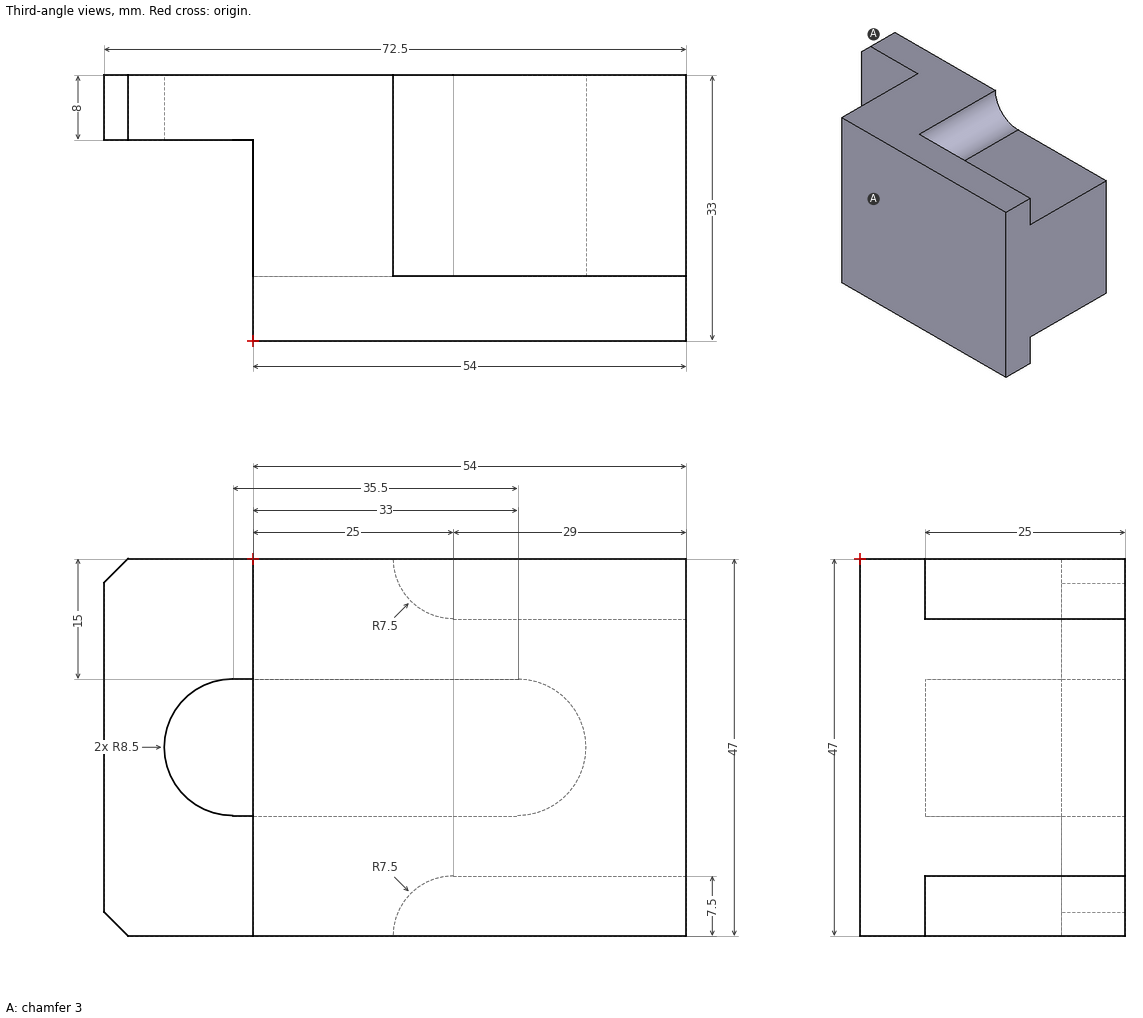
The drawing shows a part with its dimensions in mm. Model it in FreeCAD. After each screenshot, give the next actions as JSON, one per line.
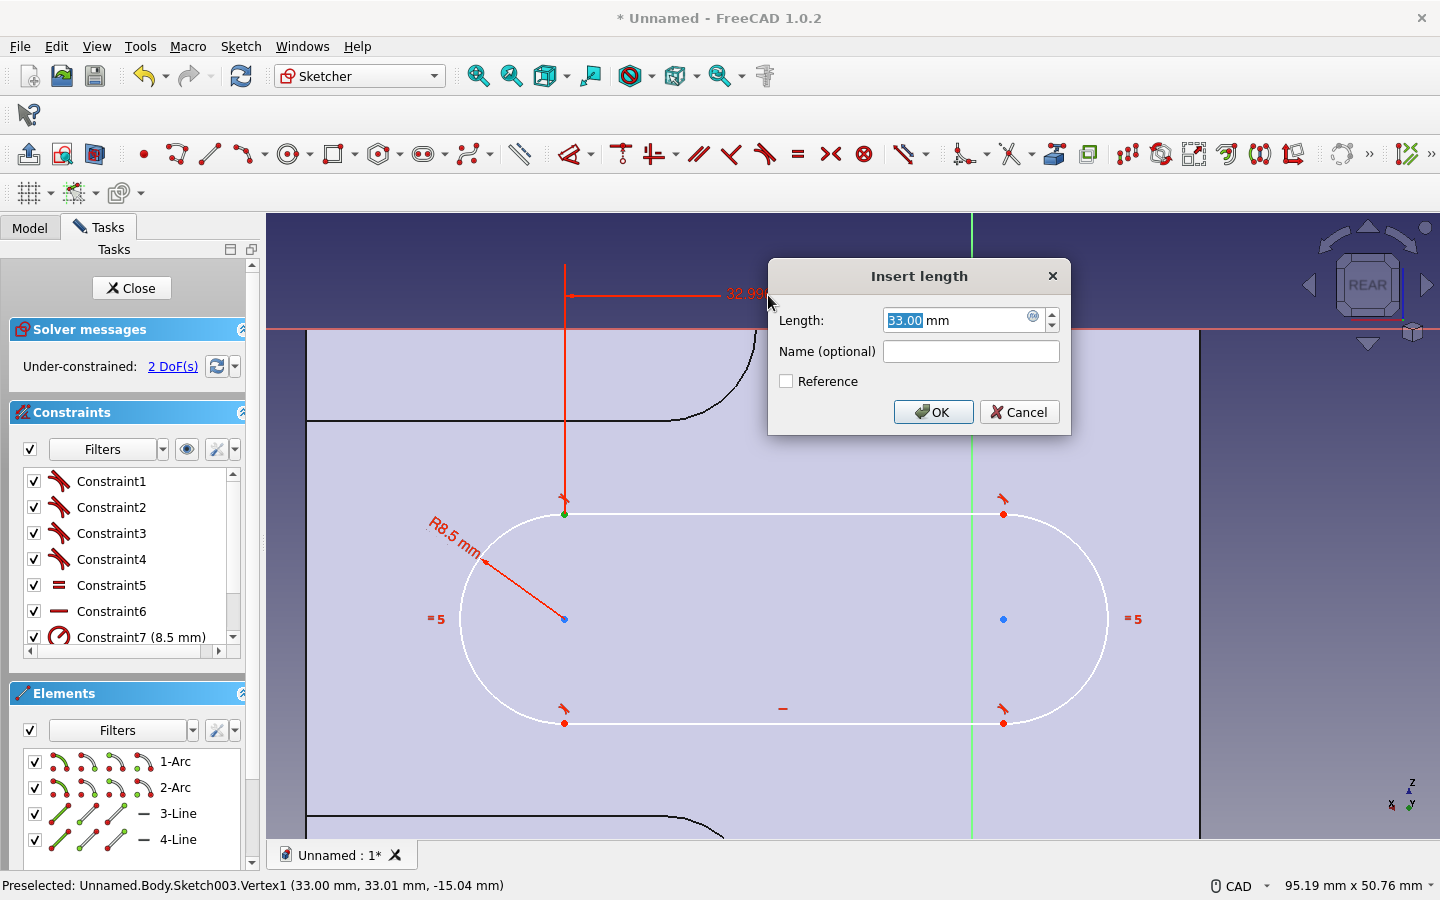
{"action": "type", "text": "33"}
{"action": "key", "text": "Return"}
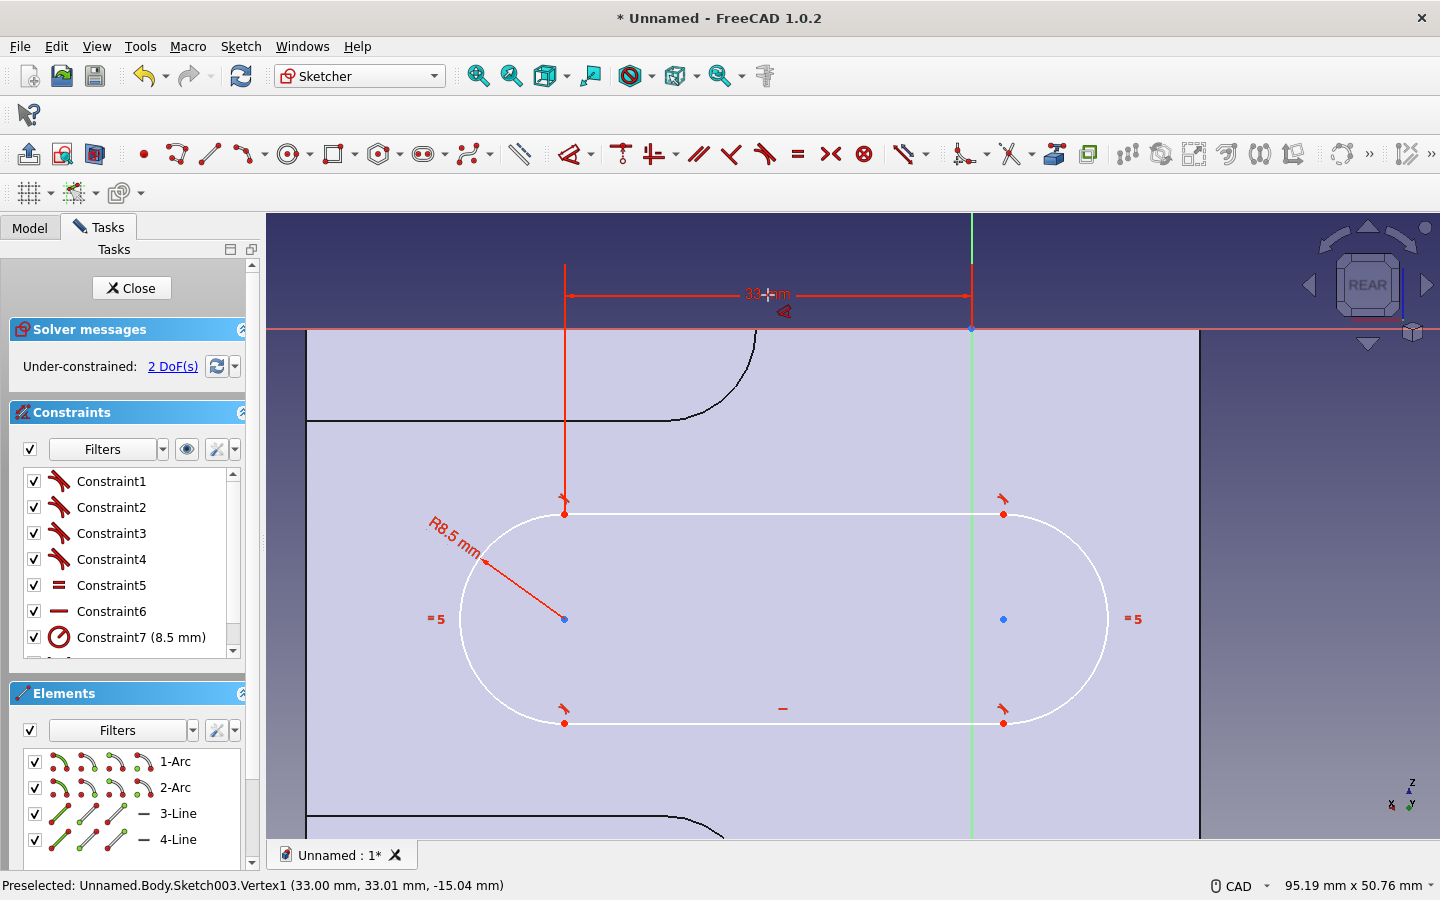
{"action": "left_click", "coordinate": [565, 514]}
{"action": "left_click", "coordinate": [531, 422]}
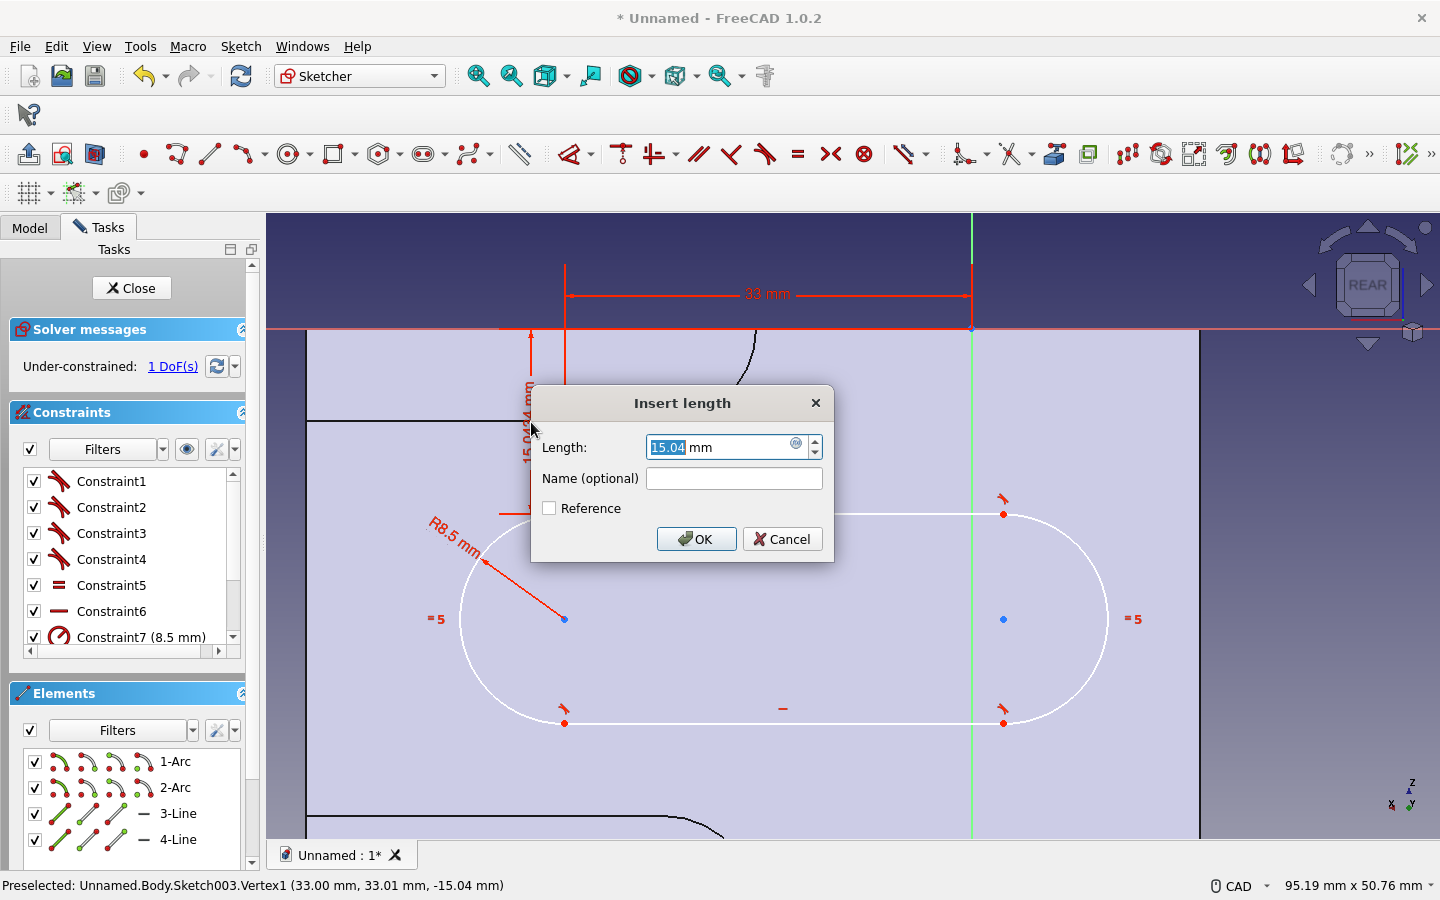
{"action": "type", "text": "15"}
{"action": "key", "text": "Return"}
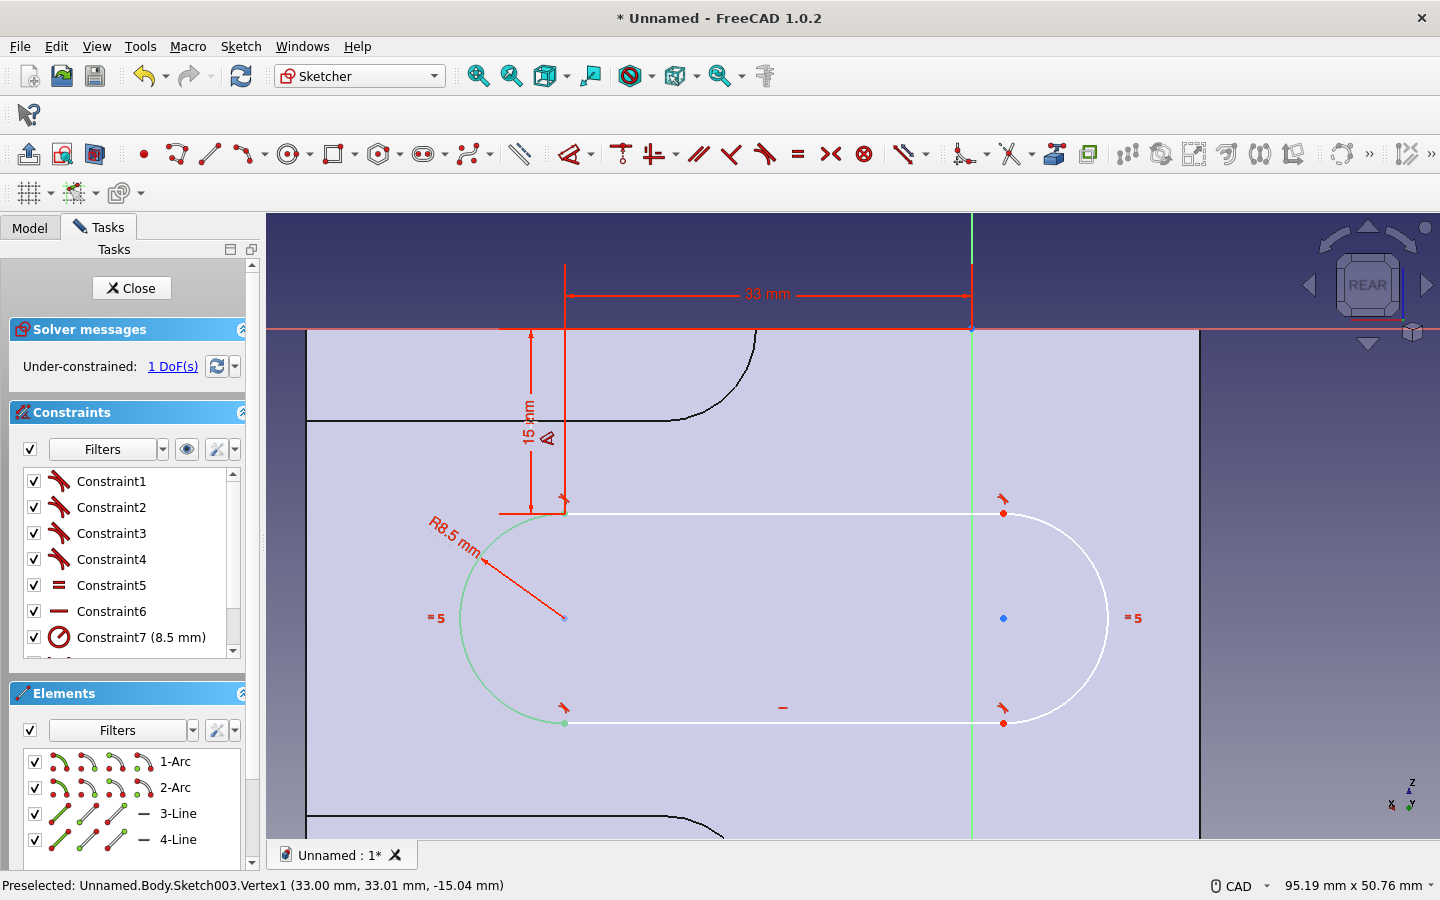
{"action": "left_click", "coordinate": [696, 514]}
{"action": "left_click", "coordinate": [784, 480]}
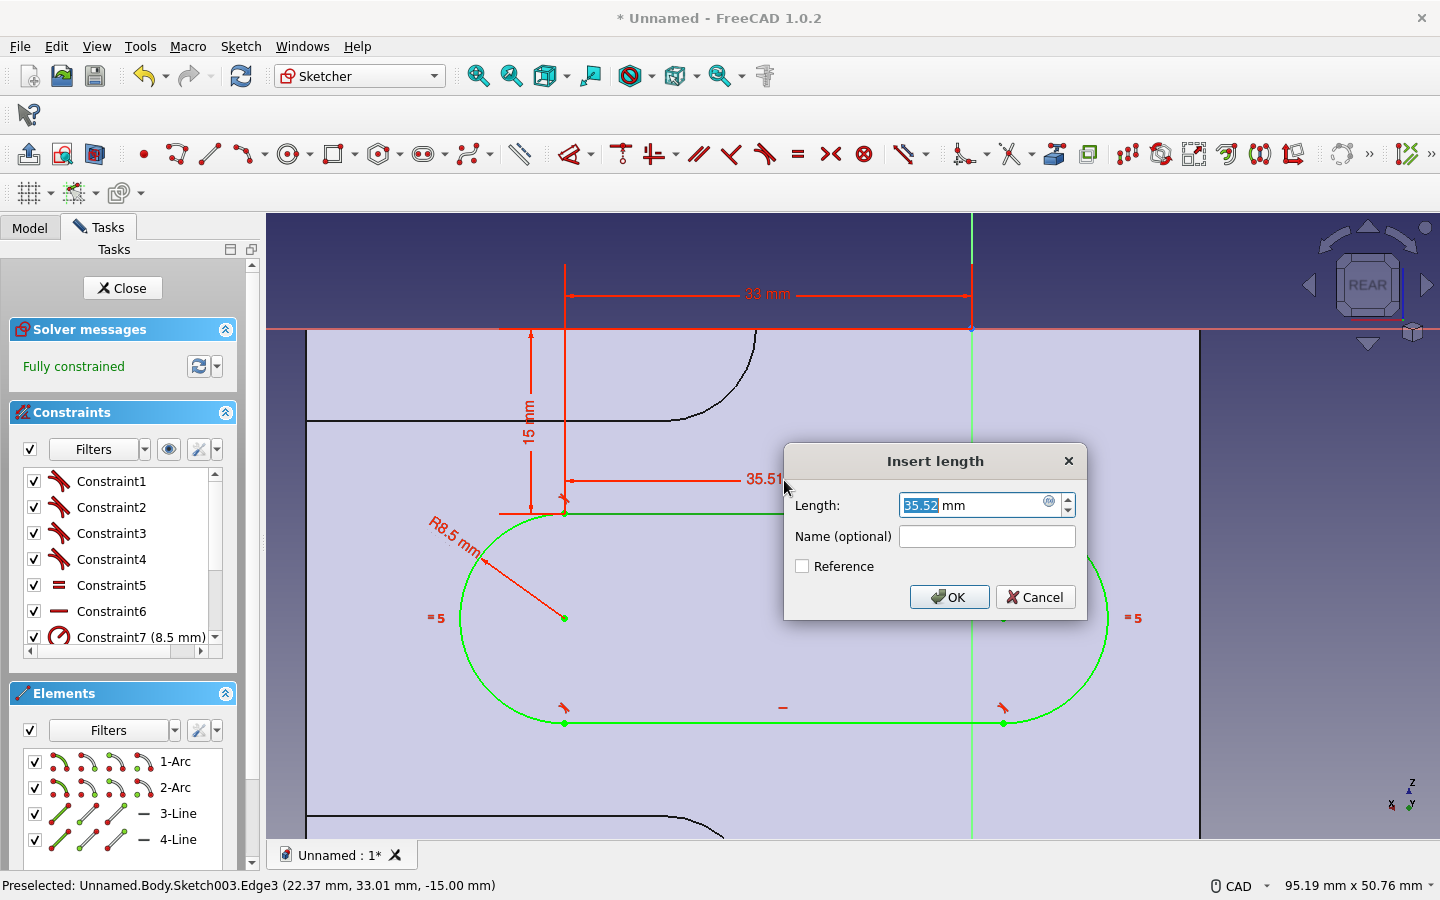
{"action": "type", "text": "35.5"}
{"action": "key", "text": "Return"}
{"action": "key", "text": "Escape"}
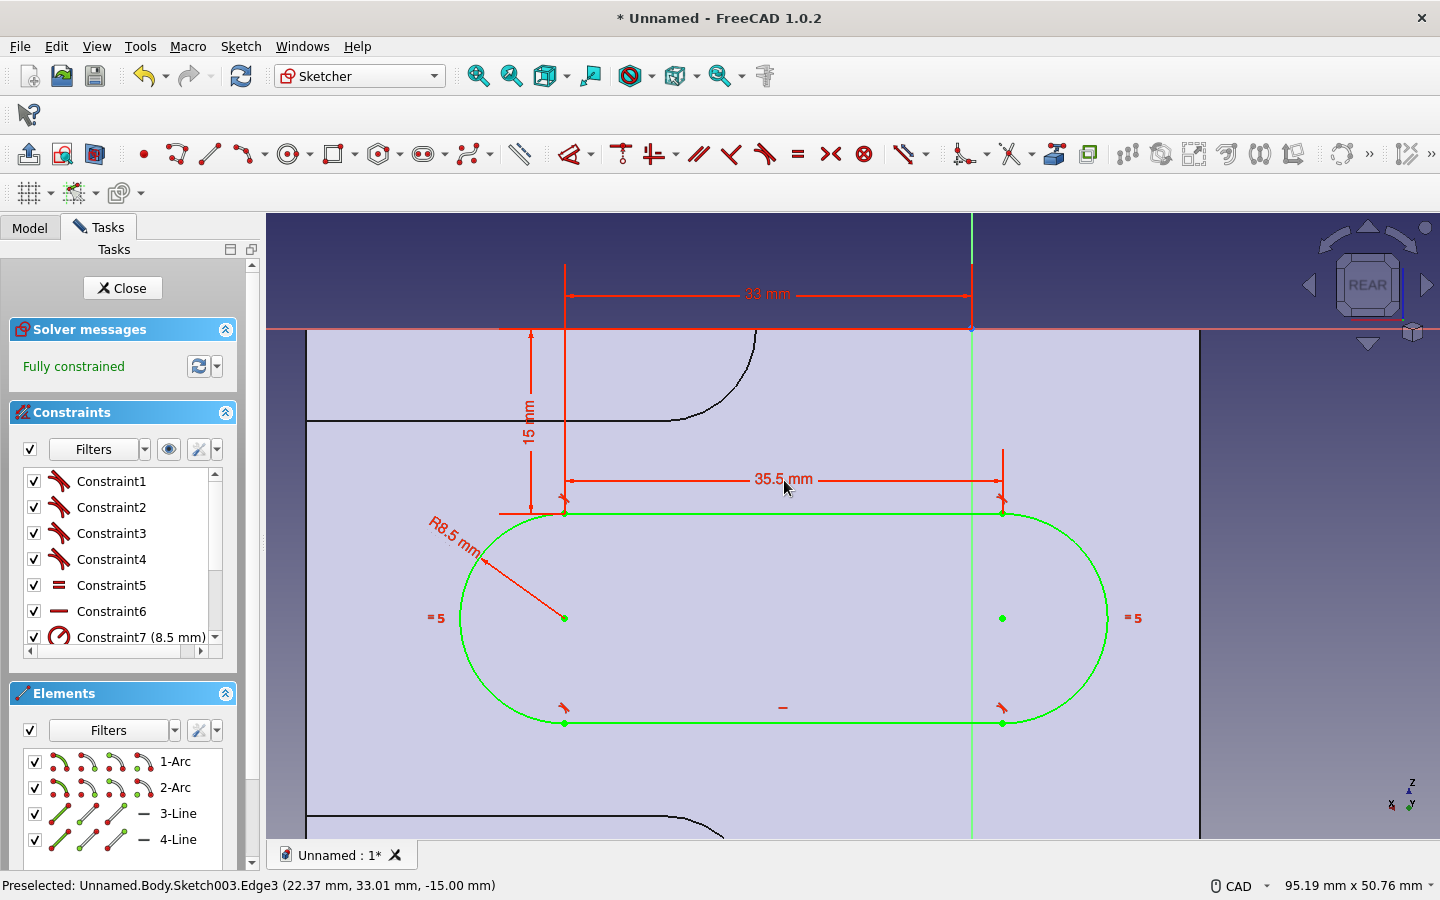
{"action": "left_click", "coordinate": [123, 288]}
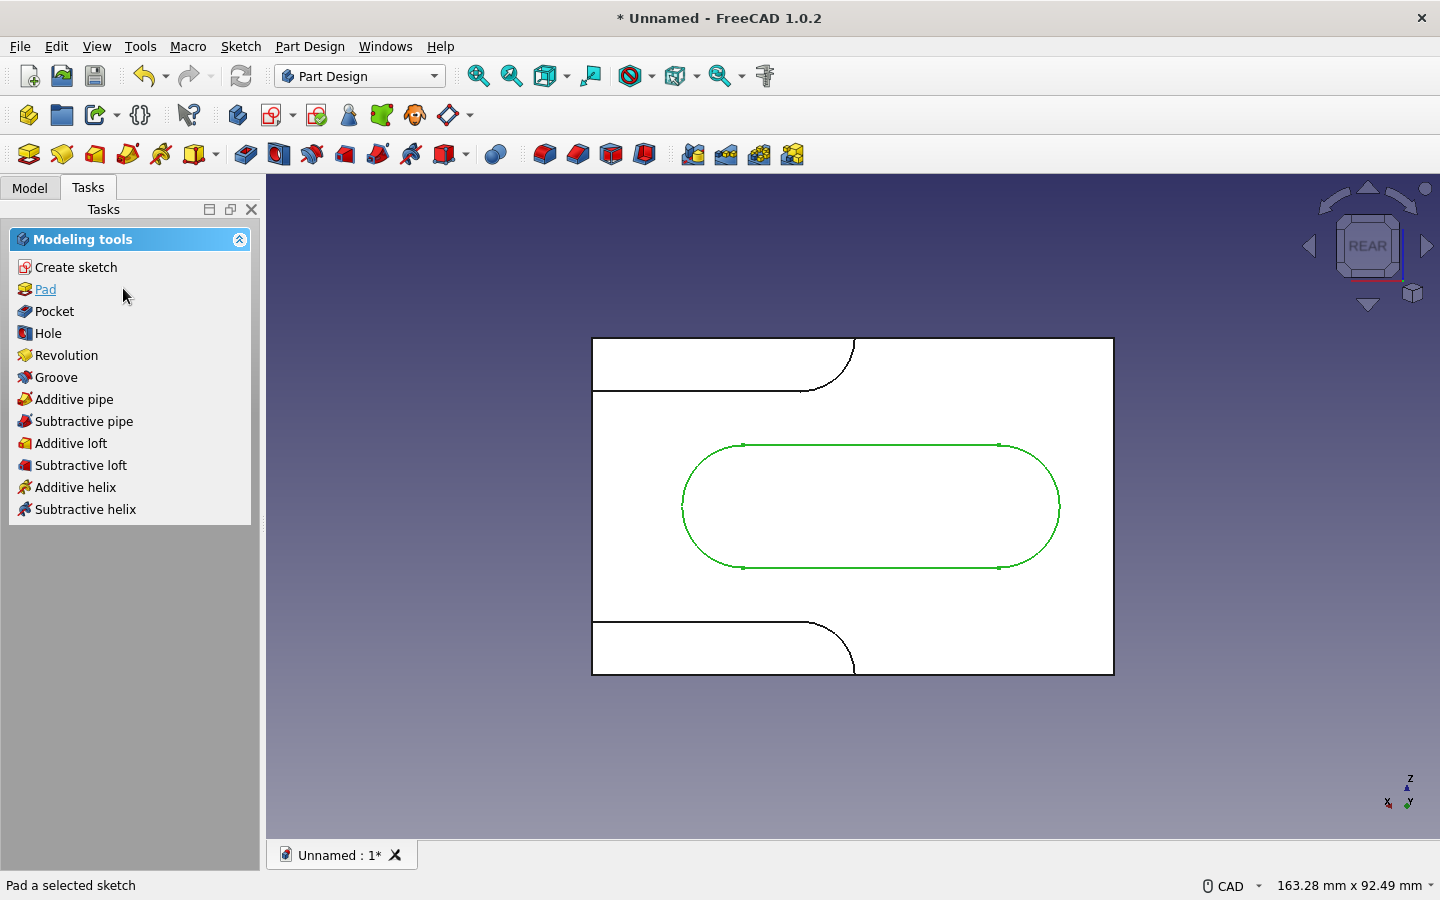
{"action": "left_click", "coordinate": [246, 154]}